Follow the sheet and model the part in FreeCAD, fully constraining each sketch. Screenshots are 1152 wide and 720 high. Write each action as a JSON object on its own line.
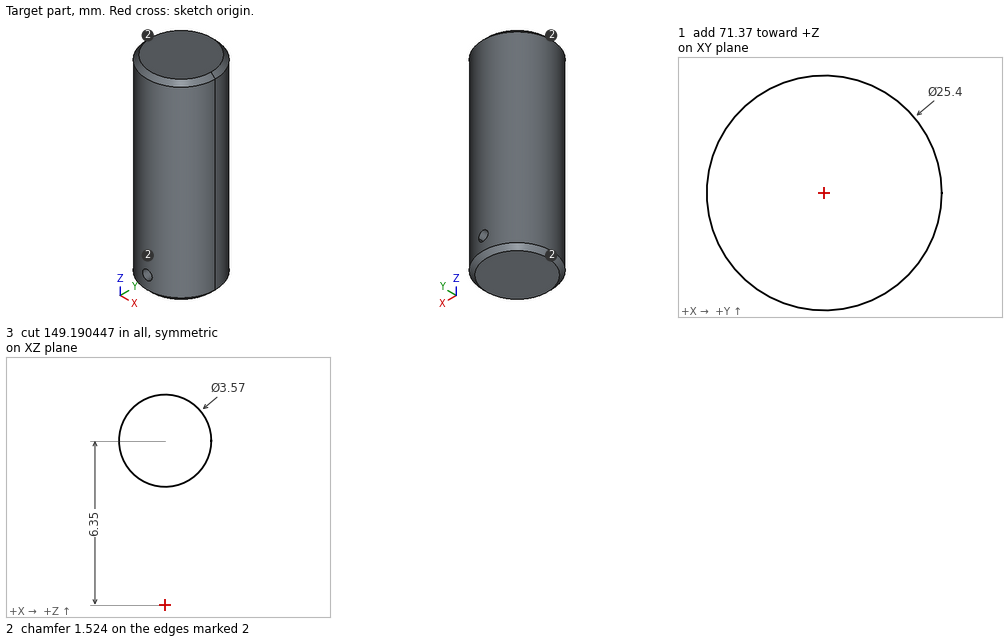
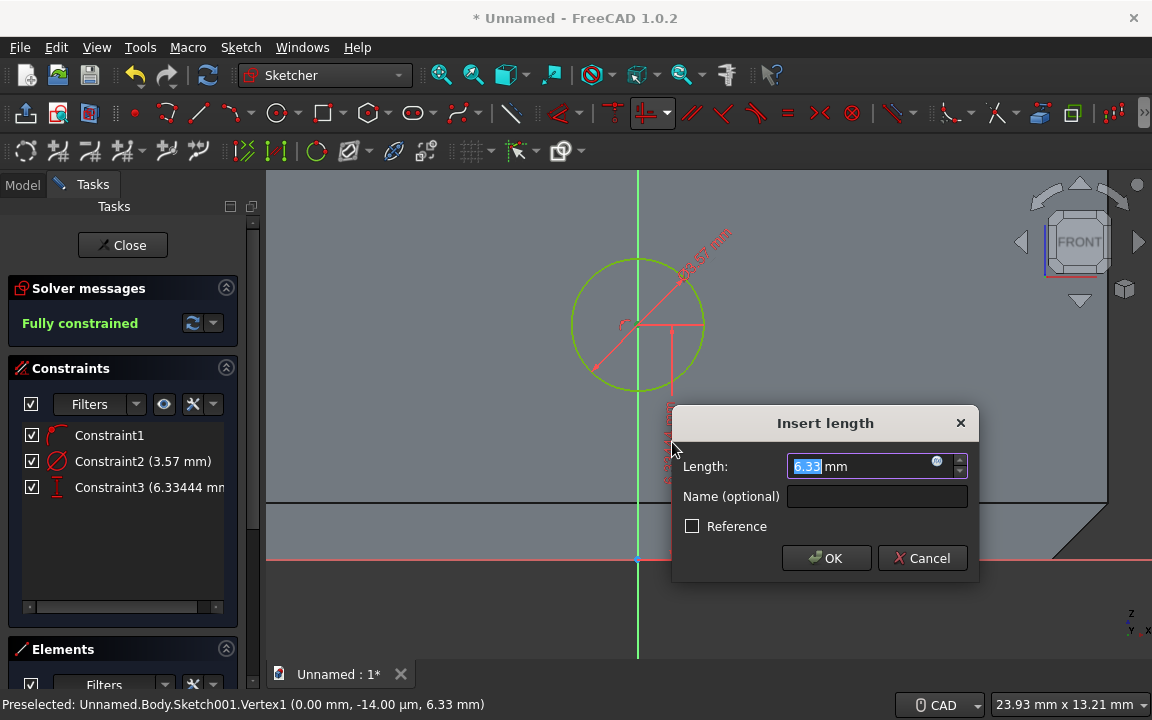
{"action": "type", "text": "6.35"}
{"action": "key", "text": "Return"}
{"action": "key", "text": "Escape"}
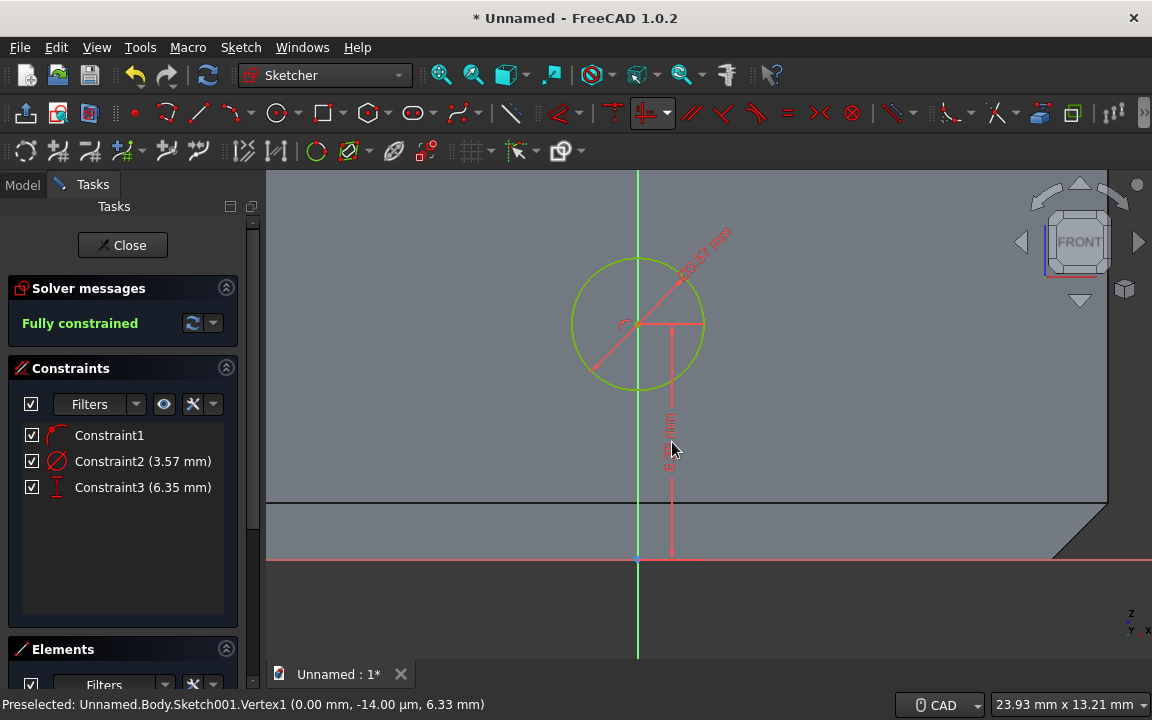
{"action": "left_click", "coordinate": [123, 245]}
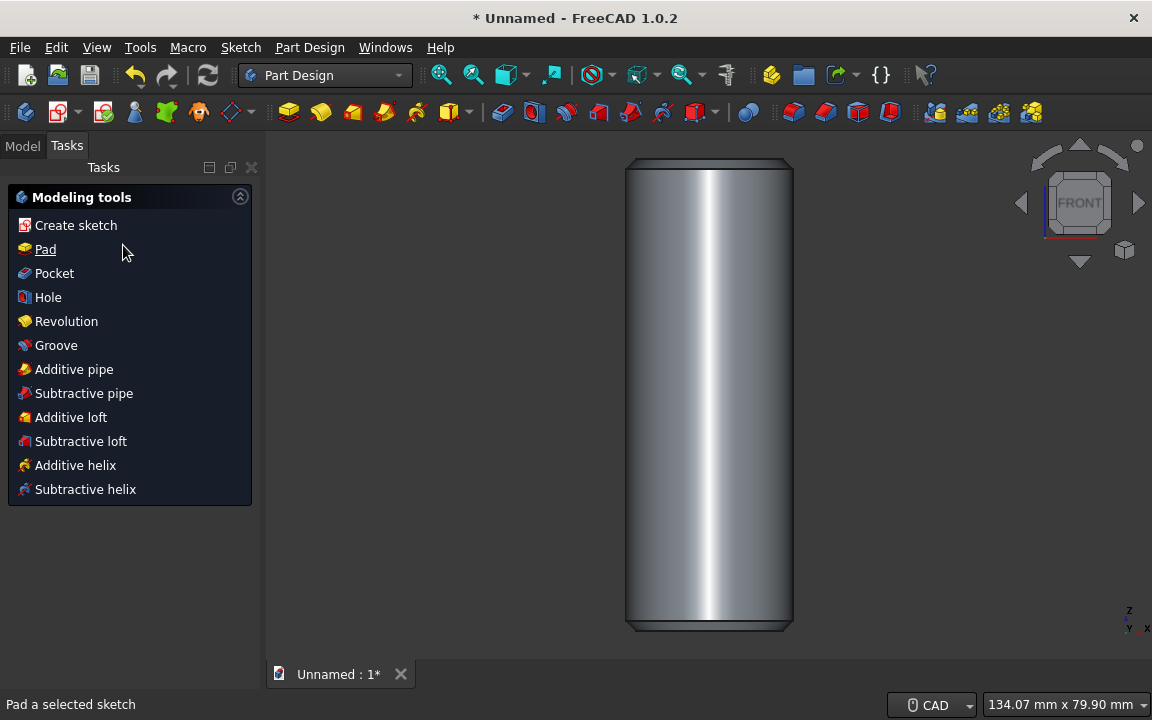
{"action": "left_click", "coordinate": [504, 112]}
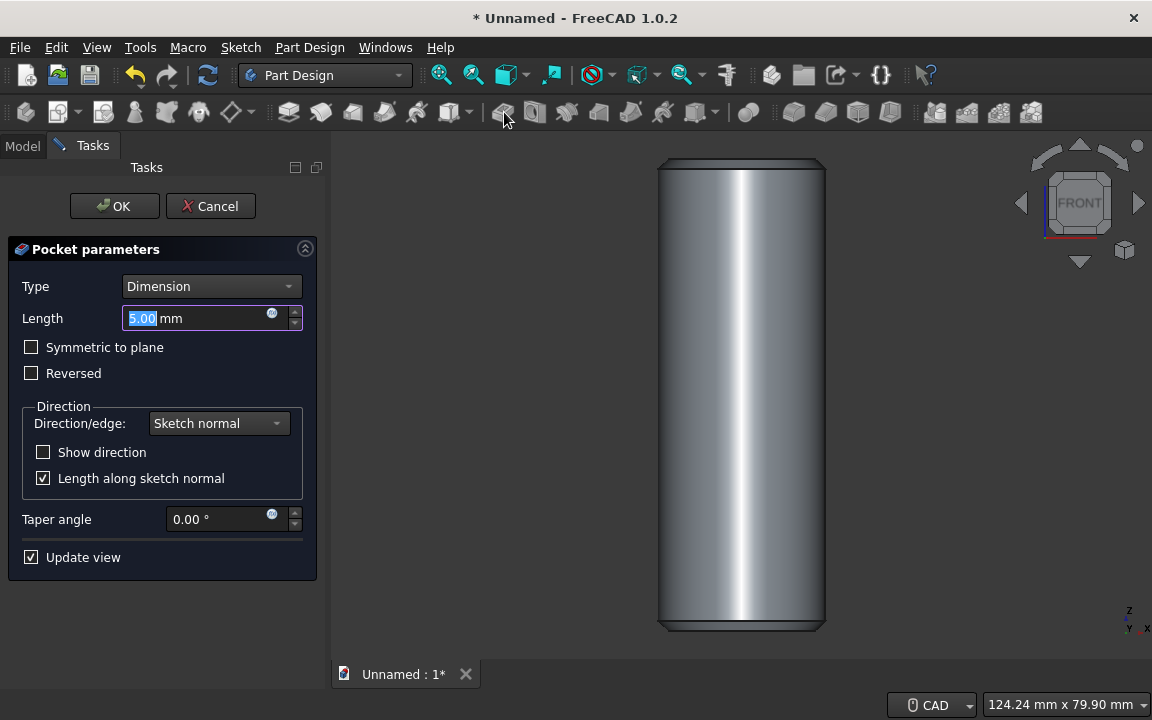
{"action": "type", "text": "149.190447"}
{"action": "key", "text": "Tab"}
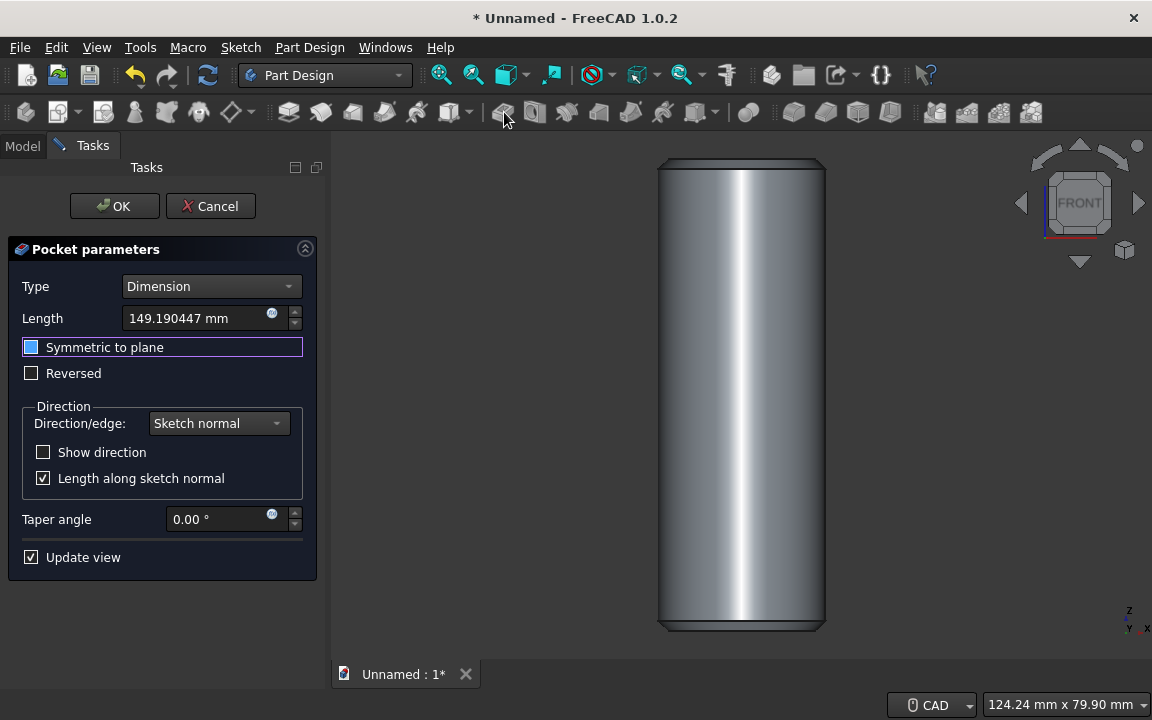
{"action": "left_click", "coordinate": [30, 347]}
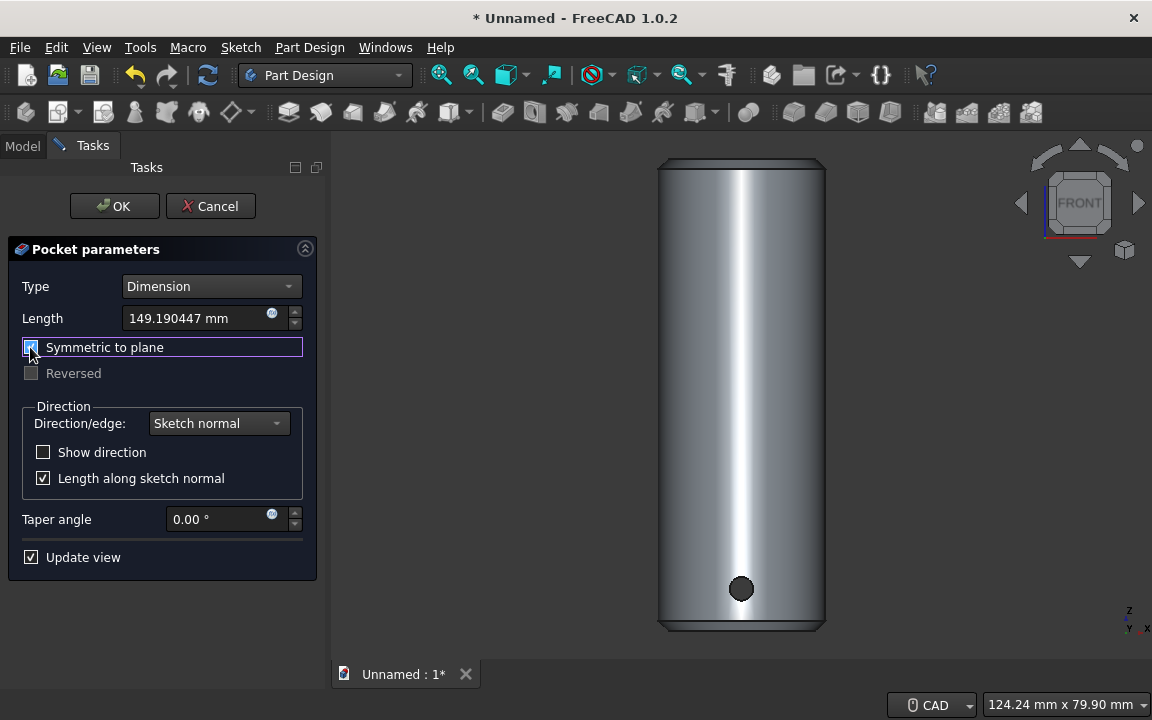
{"action": "left_click", "coordinate": [115, 206]}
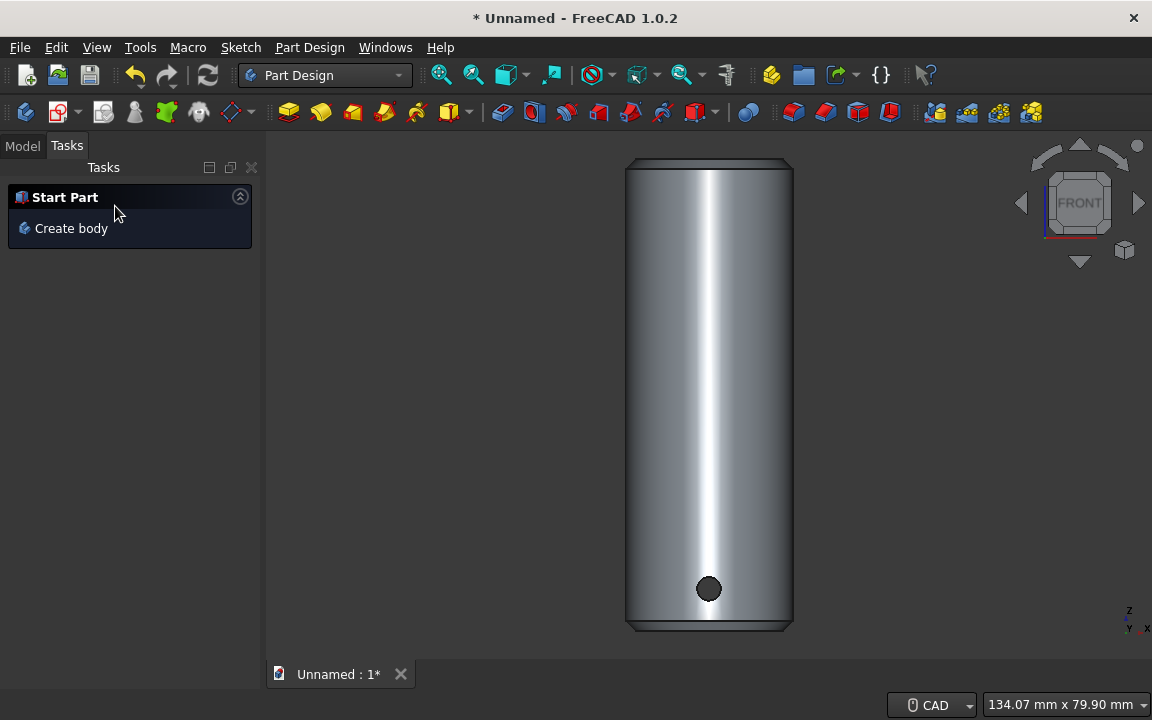
{"action": "key", "text": "0"}